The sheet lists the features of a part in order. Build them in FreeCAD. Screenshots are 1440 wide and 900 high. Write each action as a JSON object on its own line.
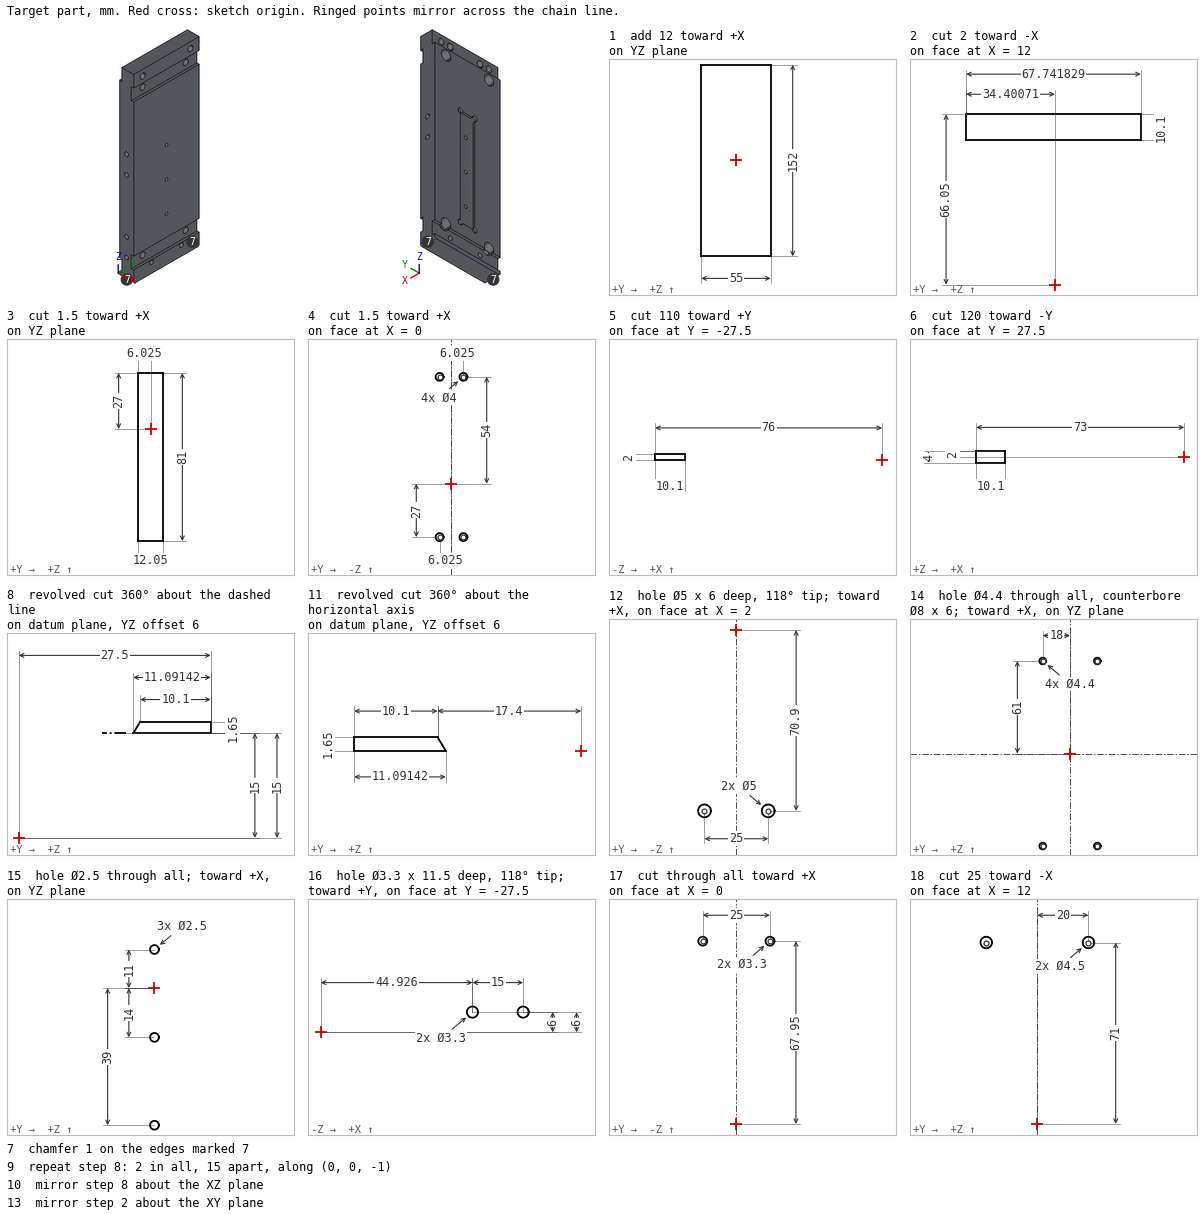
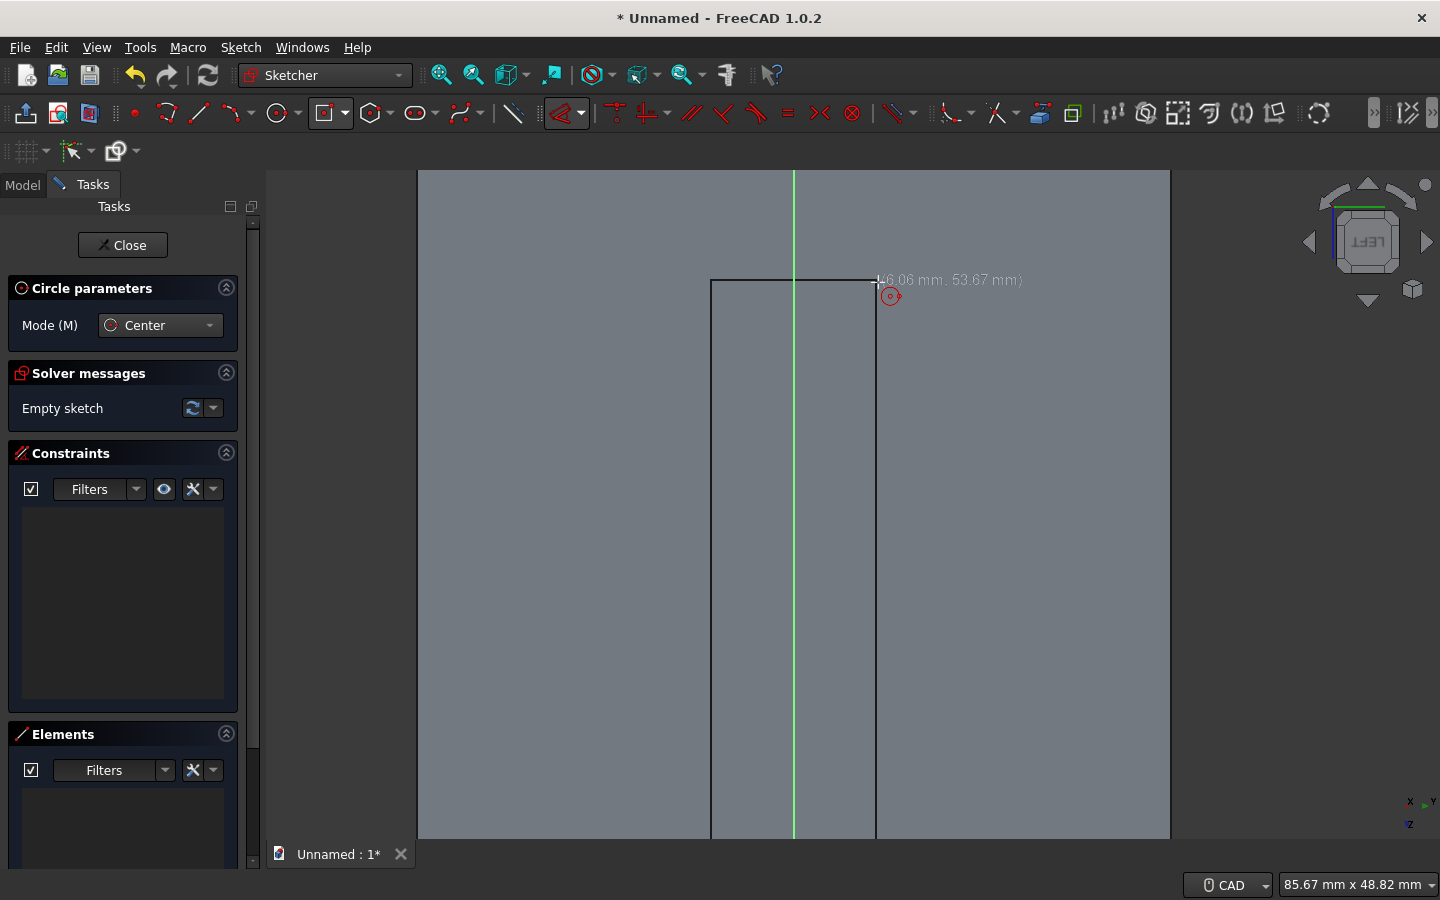
{"action": "left_click", "coordinate": [876, 280]}
{"action": "mouse_move", "coordinate": [896, 261]}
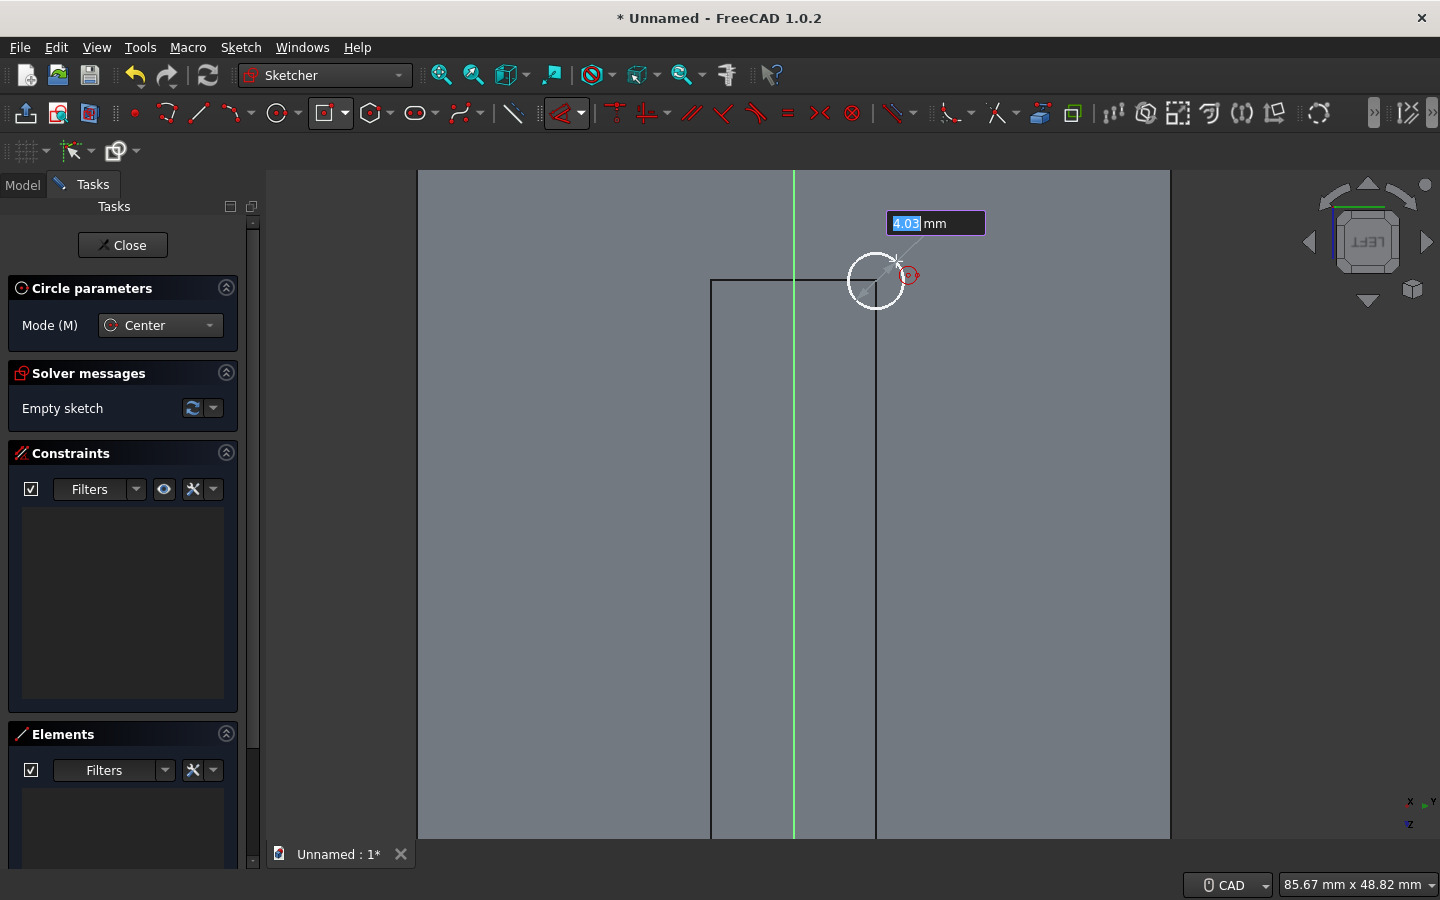
{"action": "type", "text": "4"}
{"action": "key", "text": "Return"}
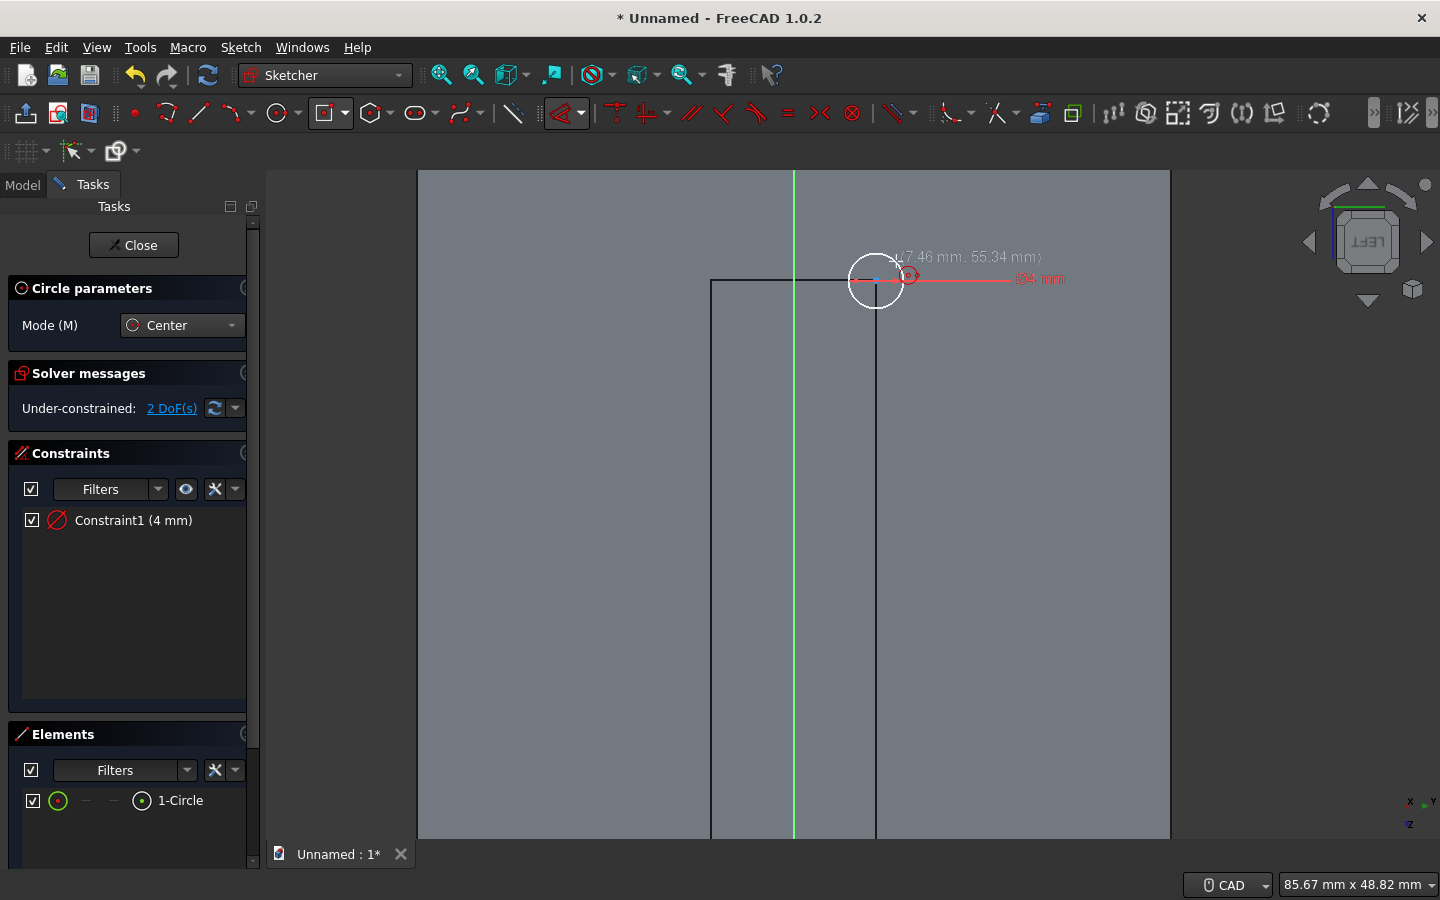
{"action": "left_click", "coordinate": [711, 280]}
{"action": "mouse_move", "coordinate": [731, 261]}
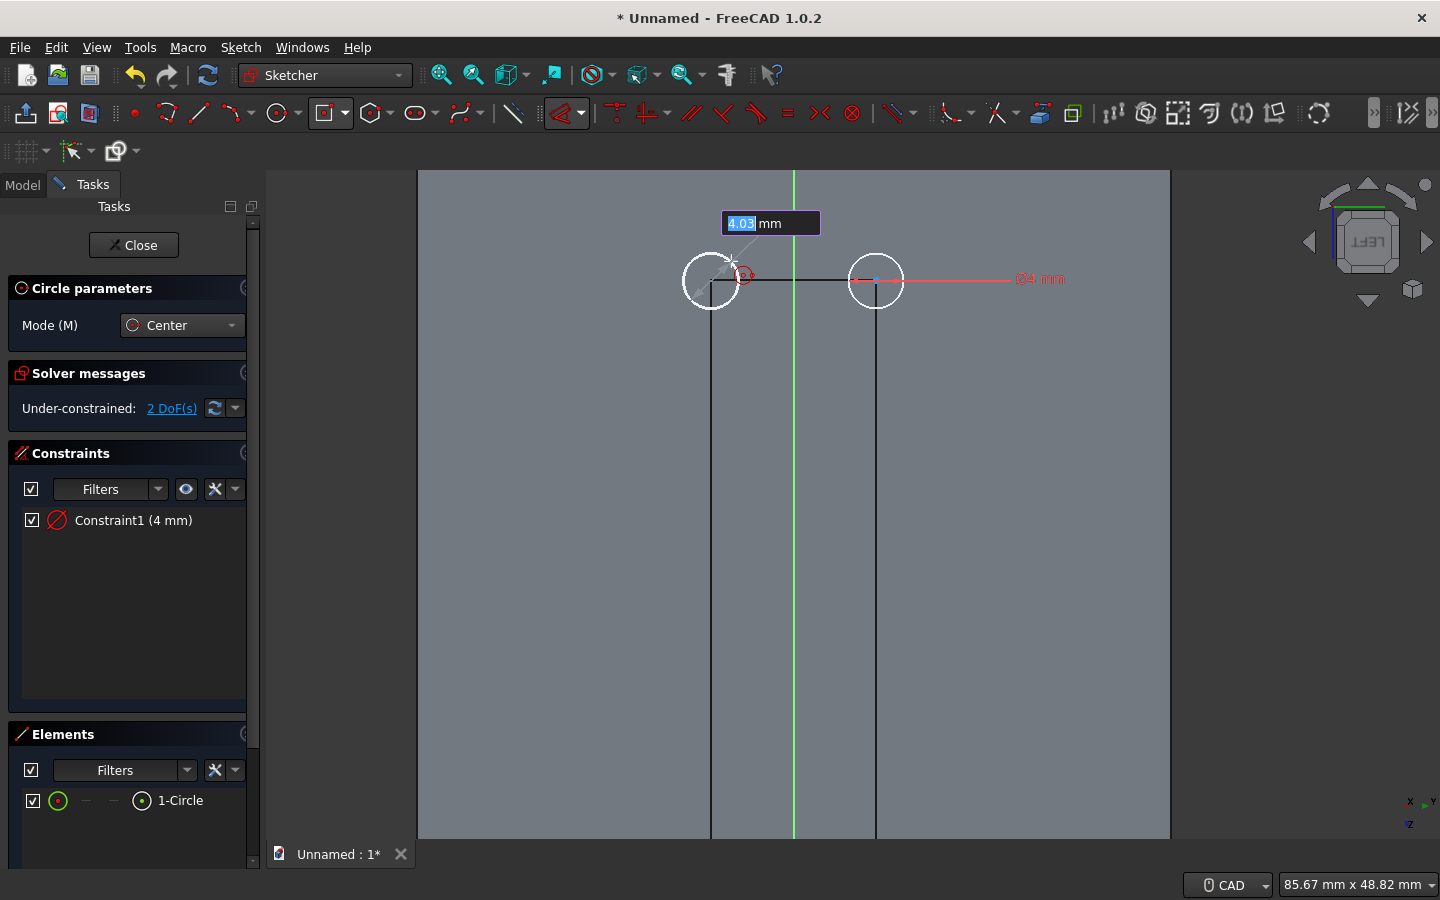
{"action": "type", "text": "4"}
{"action": "key", "text": "Return"}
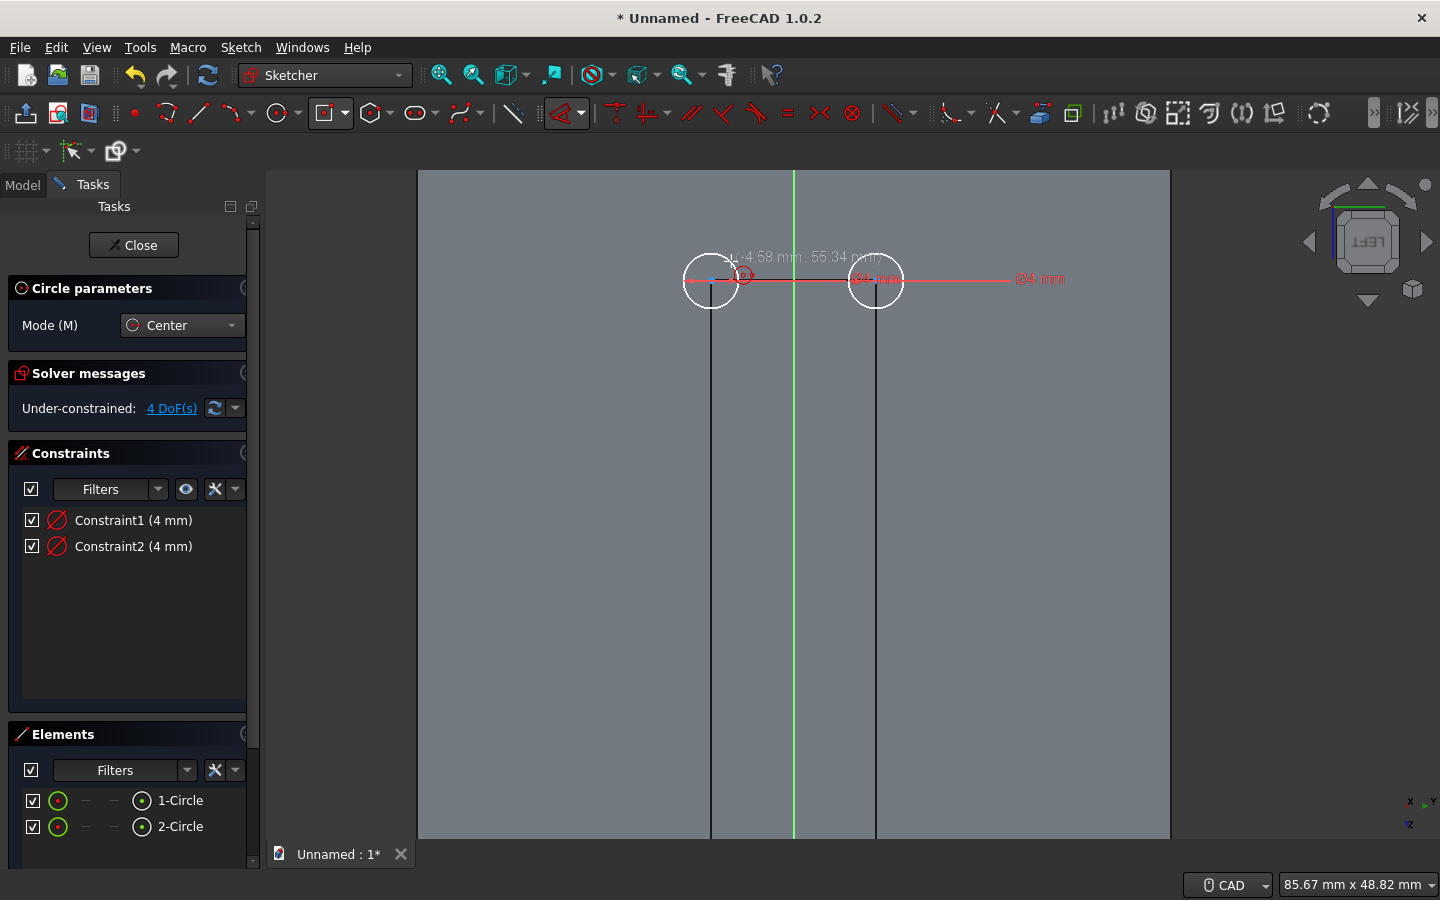
{"action": "scroll", "coordinate": [779, 312], "scroll_direction": "down", "scroll_amount": 5}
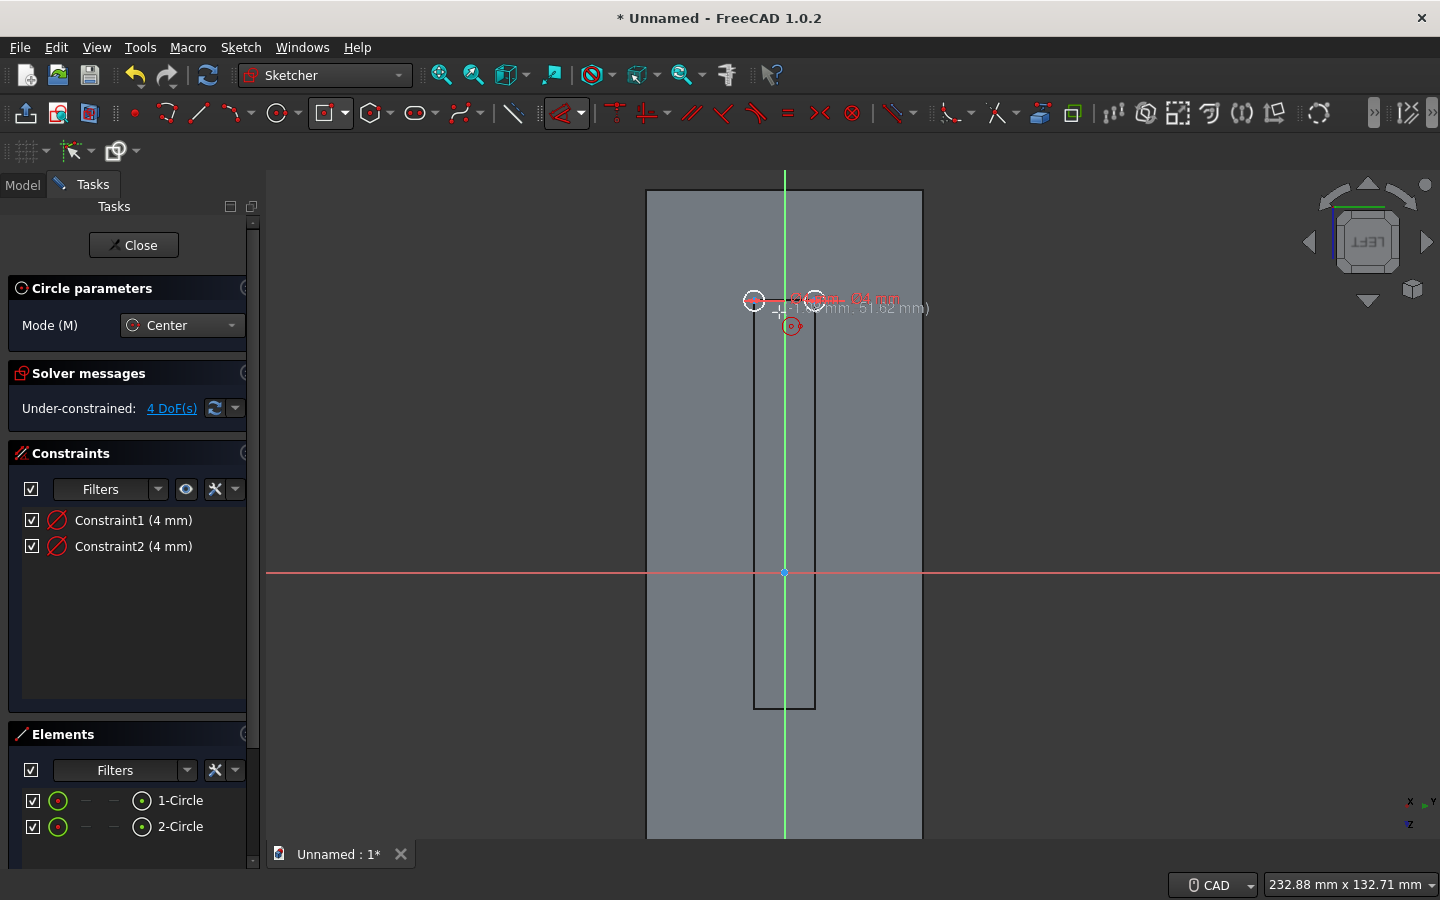
{"action": "scroll", "coordinate": [754, 709], "scroll_direction": "up", "scroll_amount": 5}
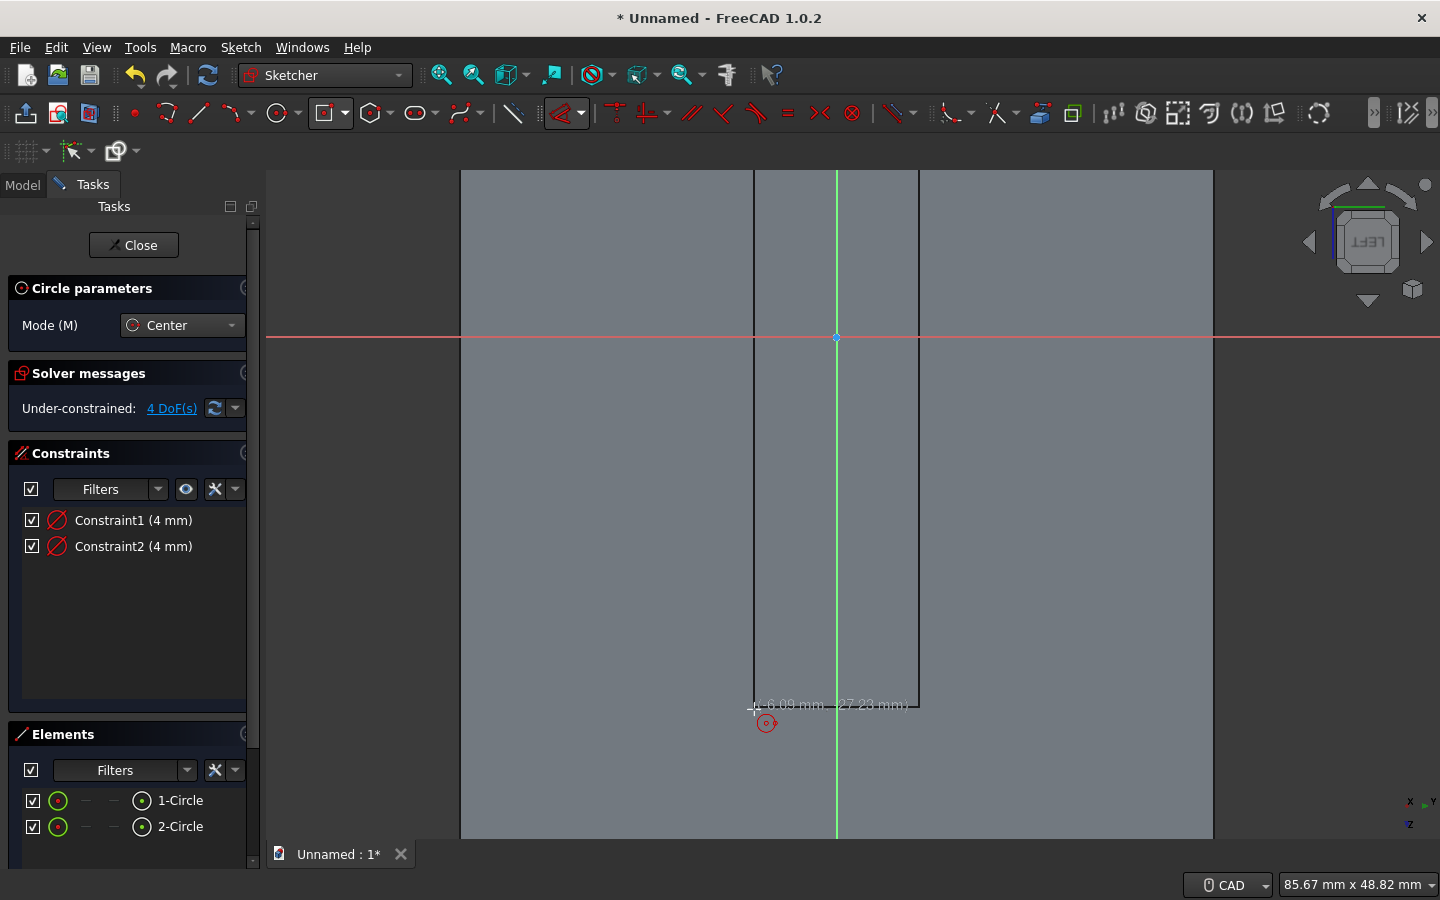
{"action": "left_click", "coordinate": [754, 707]}
{"action": "mouse_move", "coordinate": [774, 688]}